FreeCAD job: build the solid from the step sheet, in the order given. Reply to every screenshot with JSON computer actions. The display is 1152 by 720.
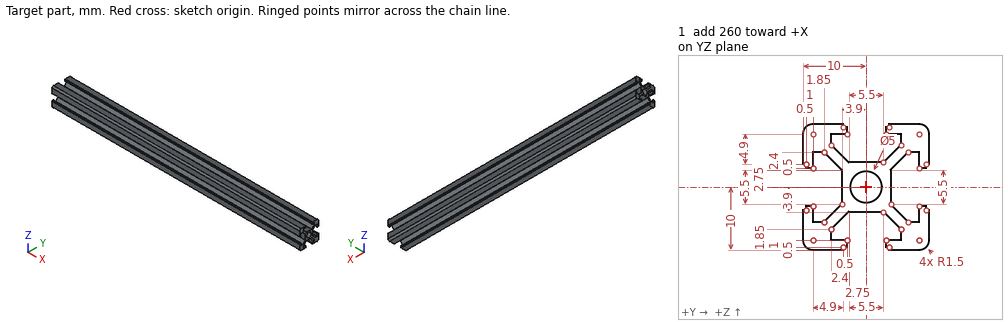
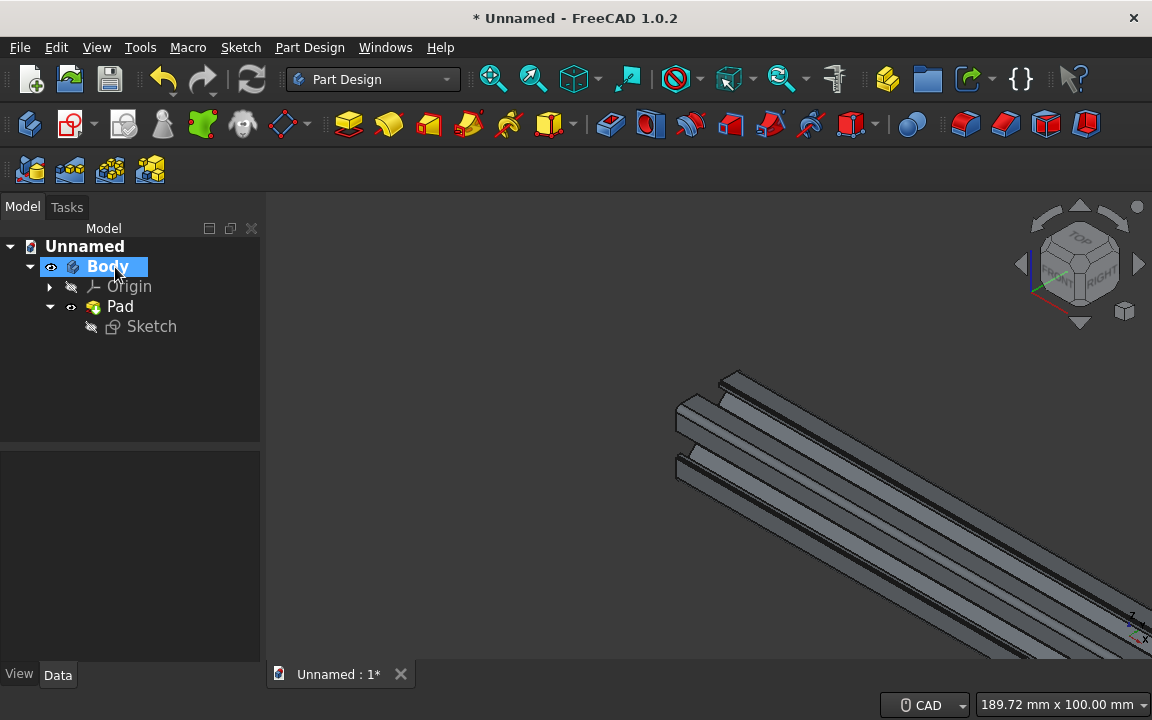
{"action": "key", "text": "v f"}